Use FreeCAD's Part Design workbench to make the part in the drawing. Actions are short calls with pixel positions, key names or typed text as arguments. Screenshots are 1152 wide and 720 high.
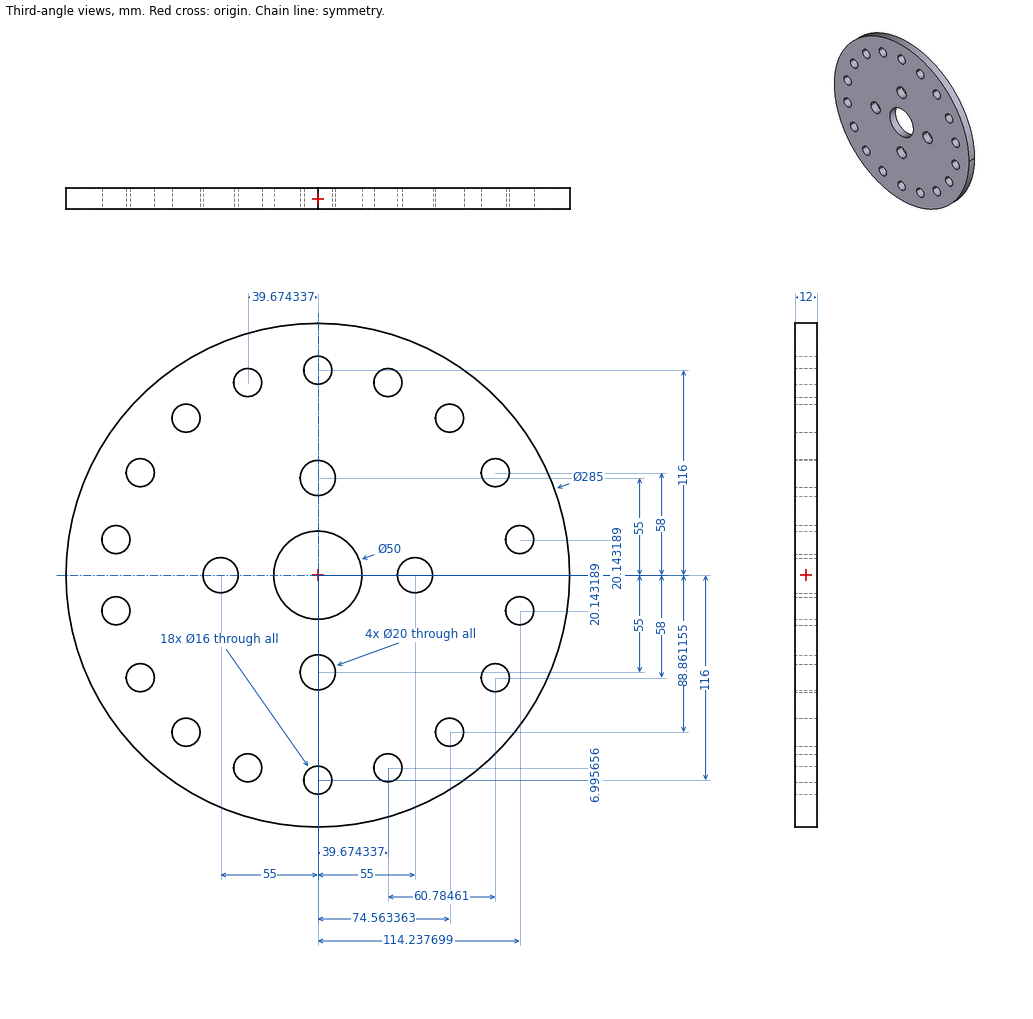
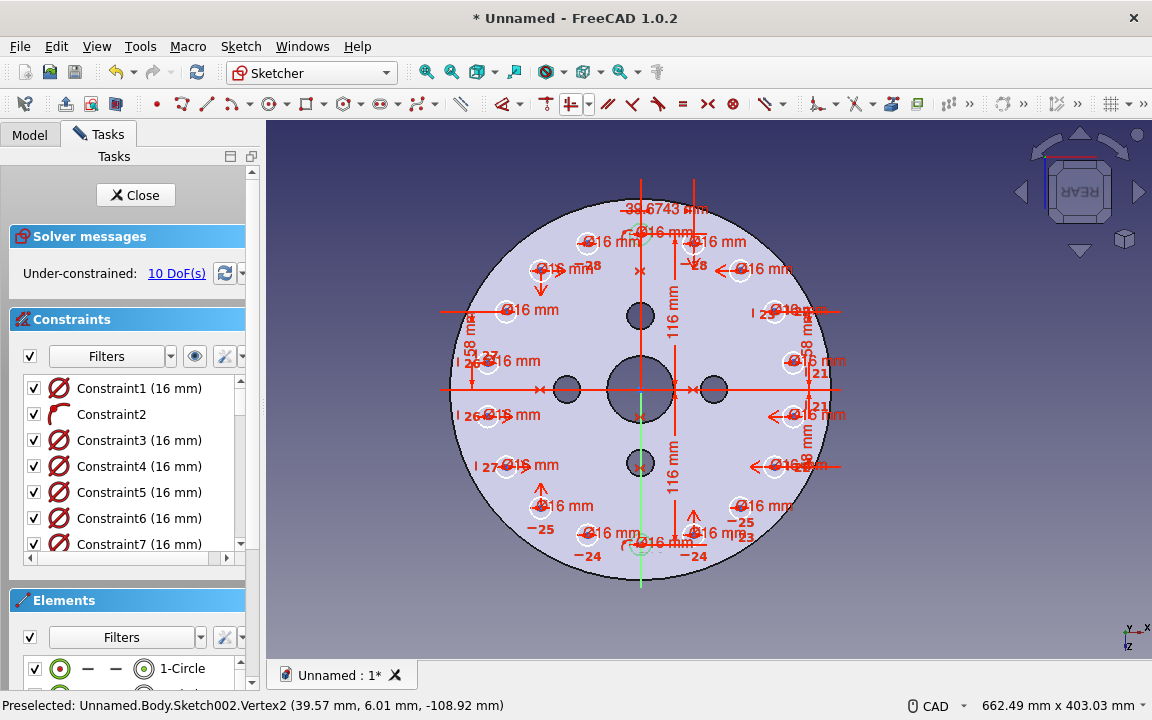
click(740, 271)
click(667, 237)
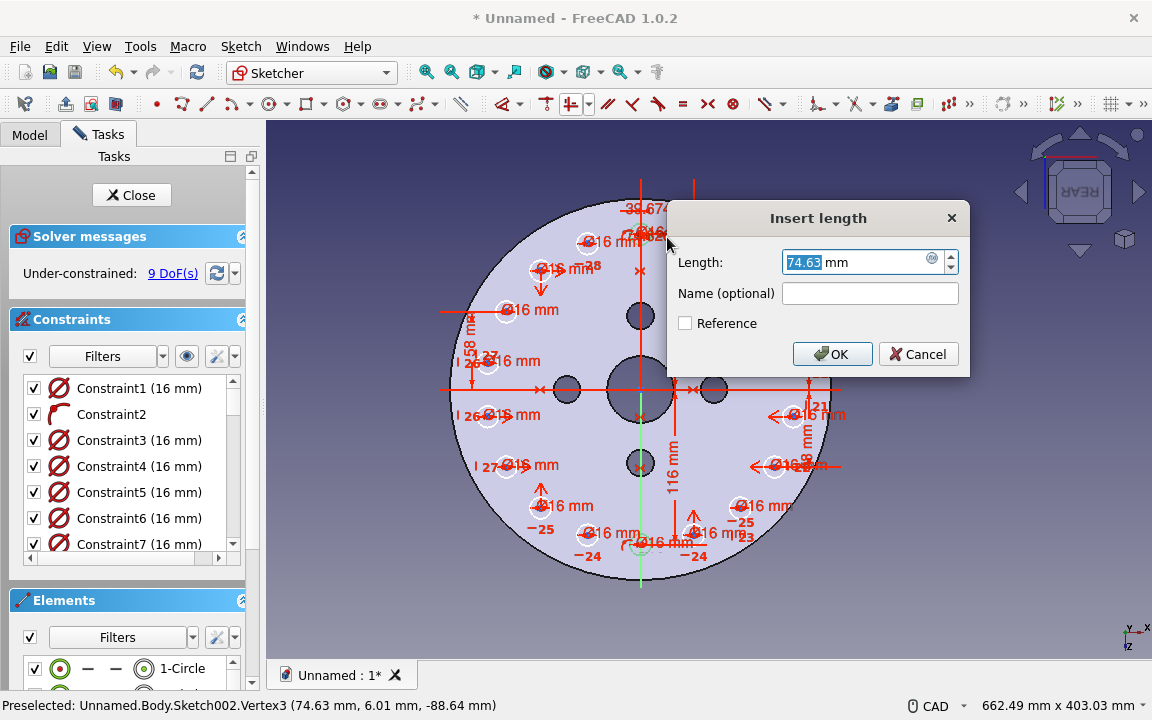
text(74.563363)
key(Return)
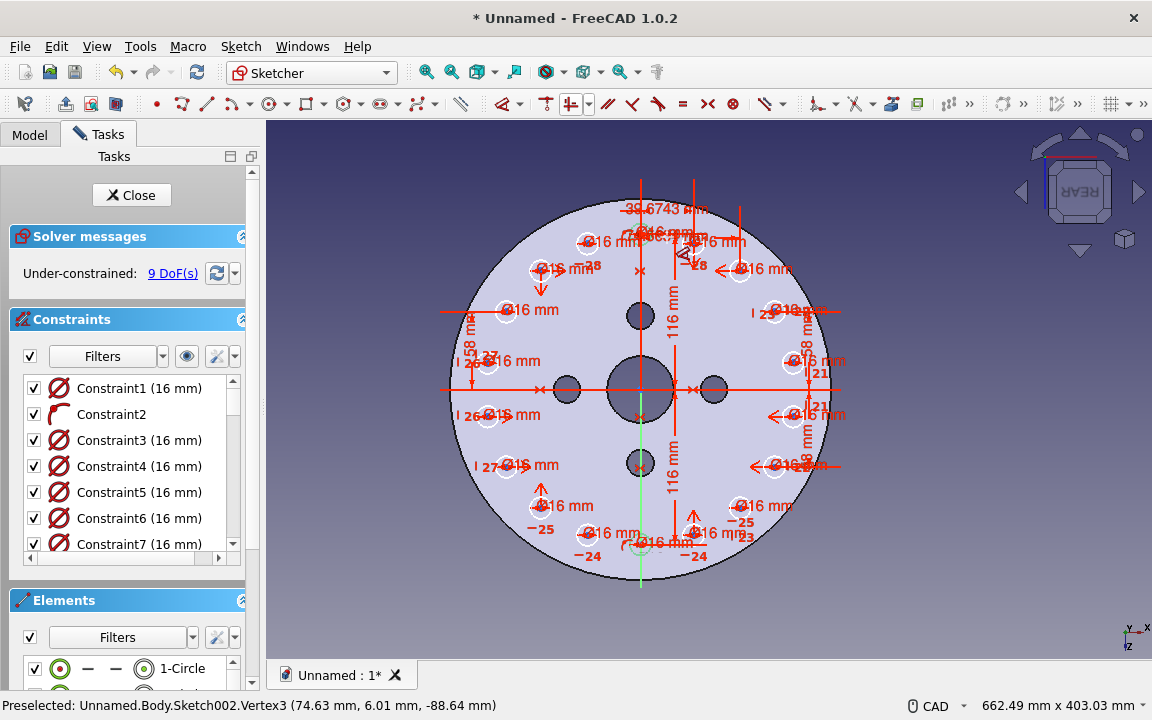
click(740, 271)
click(607, 357)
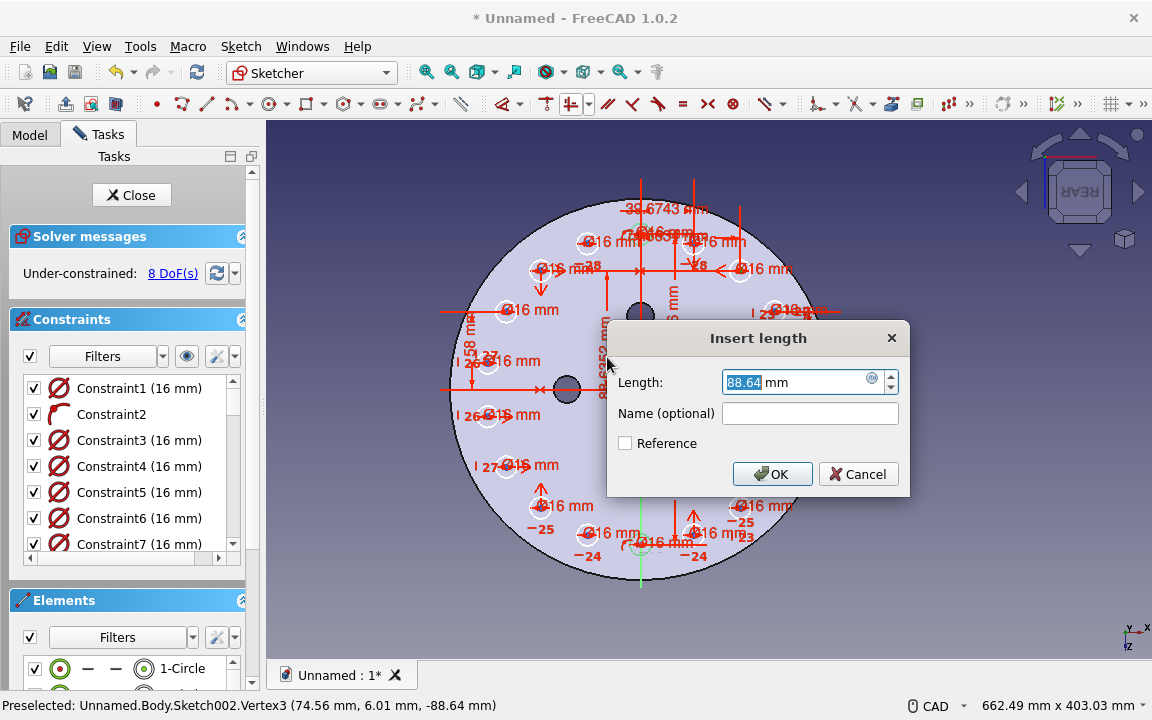
text(88.861155)
key(Return)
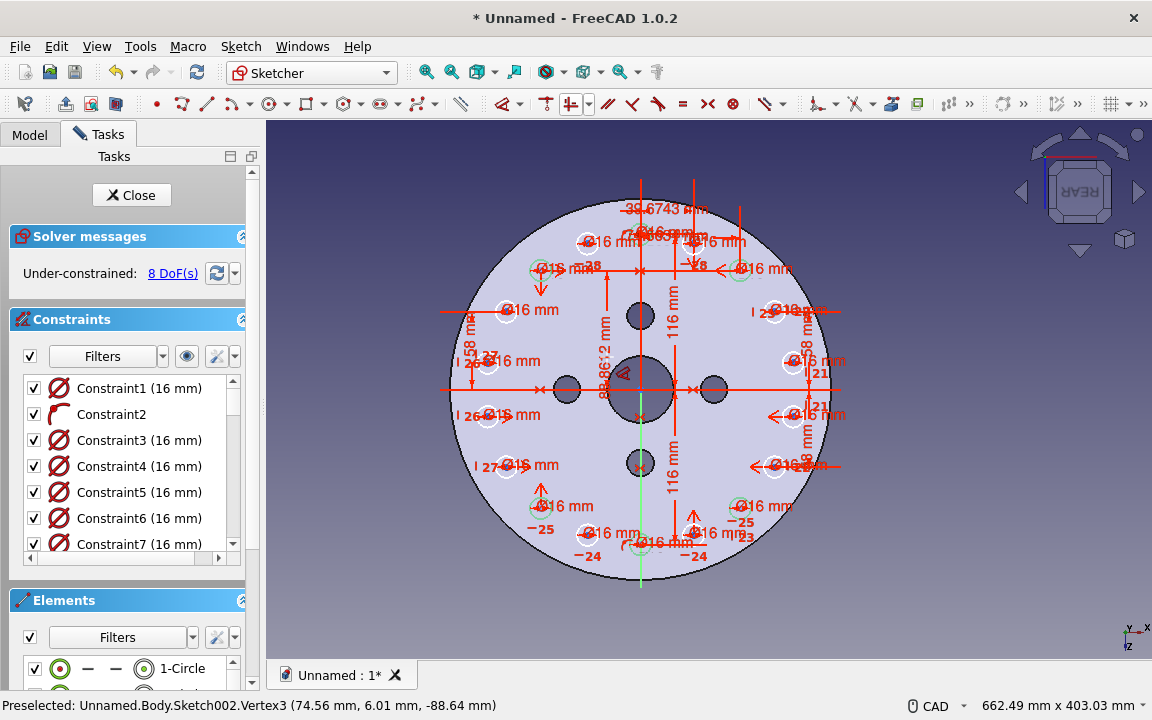
scroll(793, 363, up, 2)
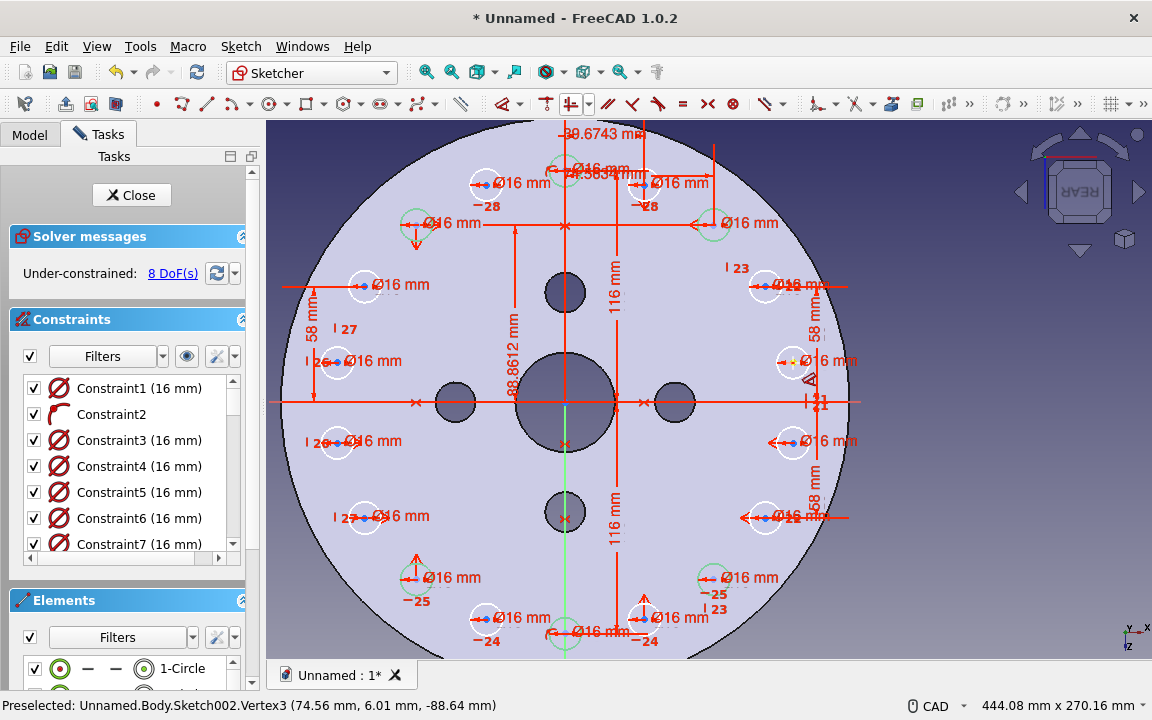
click(793, 363)
click(827, 383)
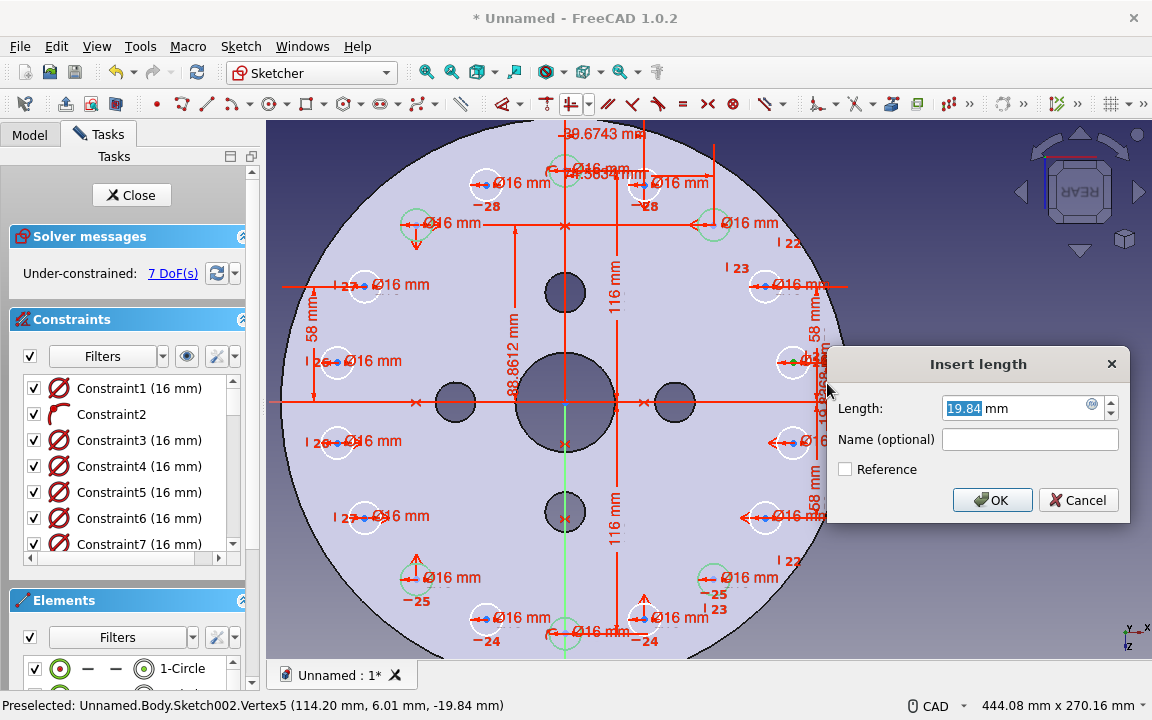
text(20.143189)
key(Return)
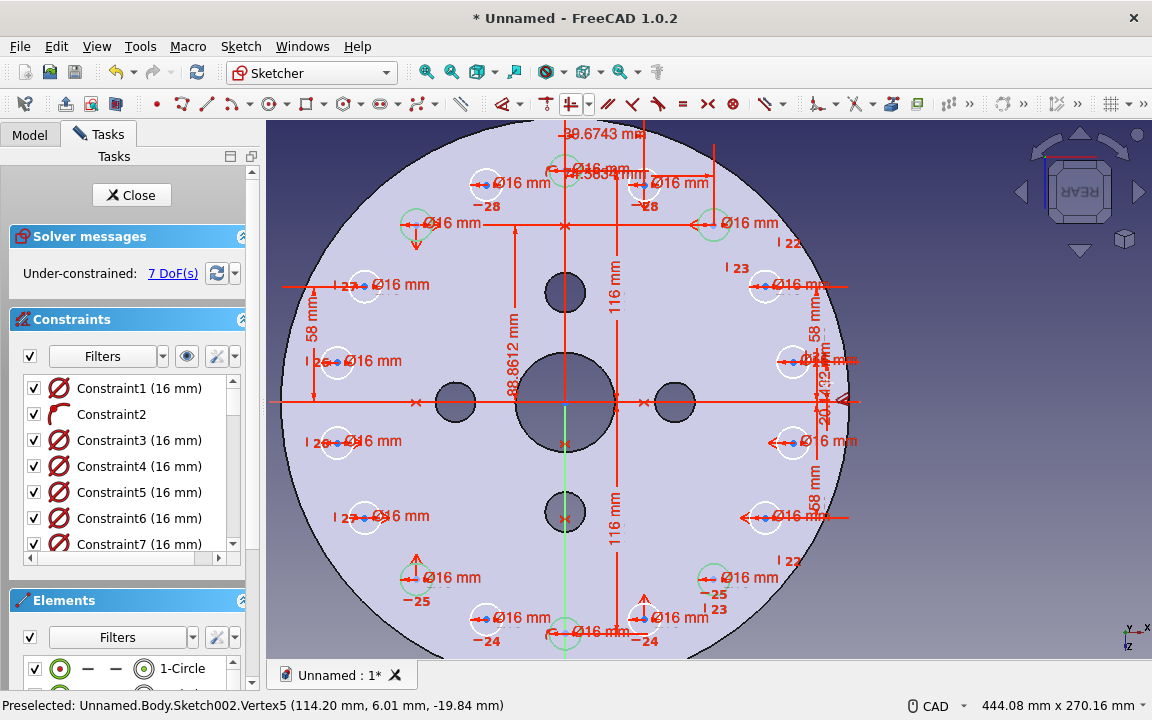
click(793, 443)
click(827, 423)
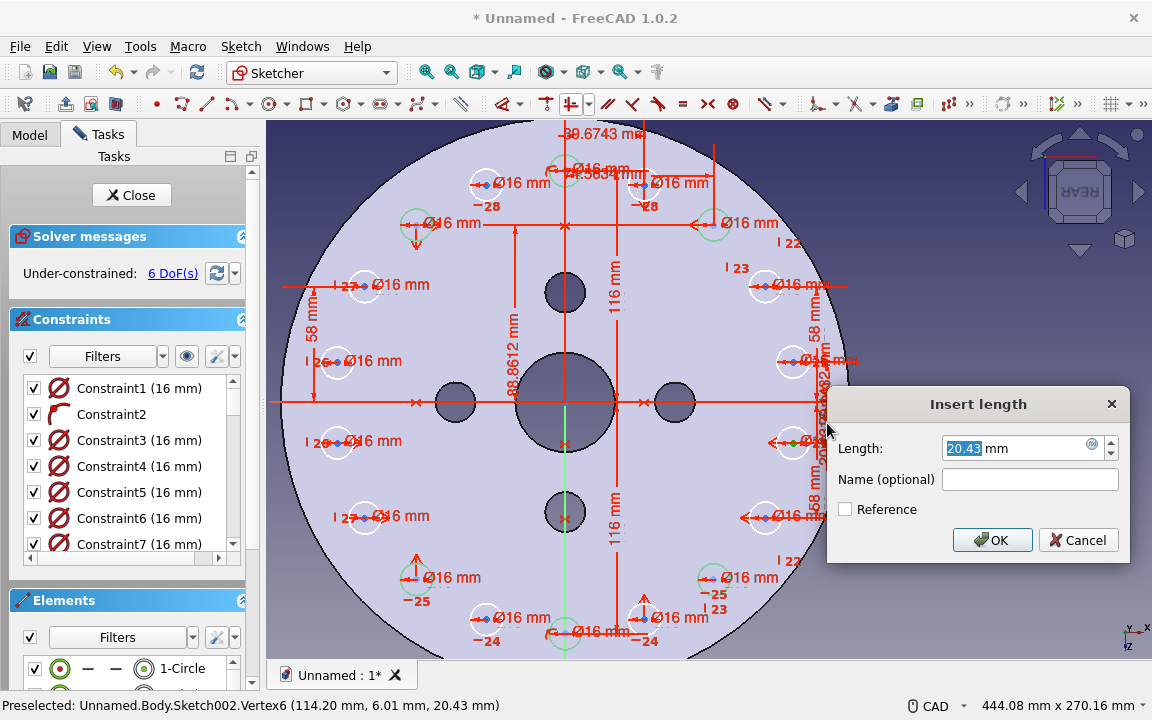
text(20.143189)
key(Return)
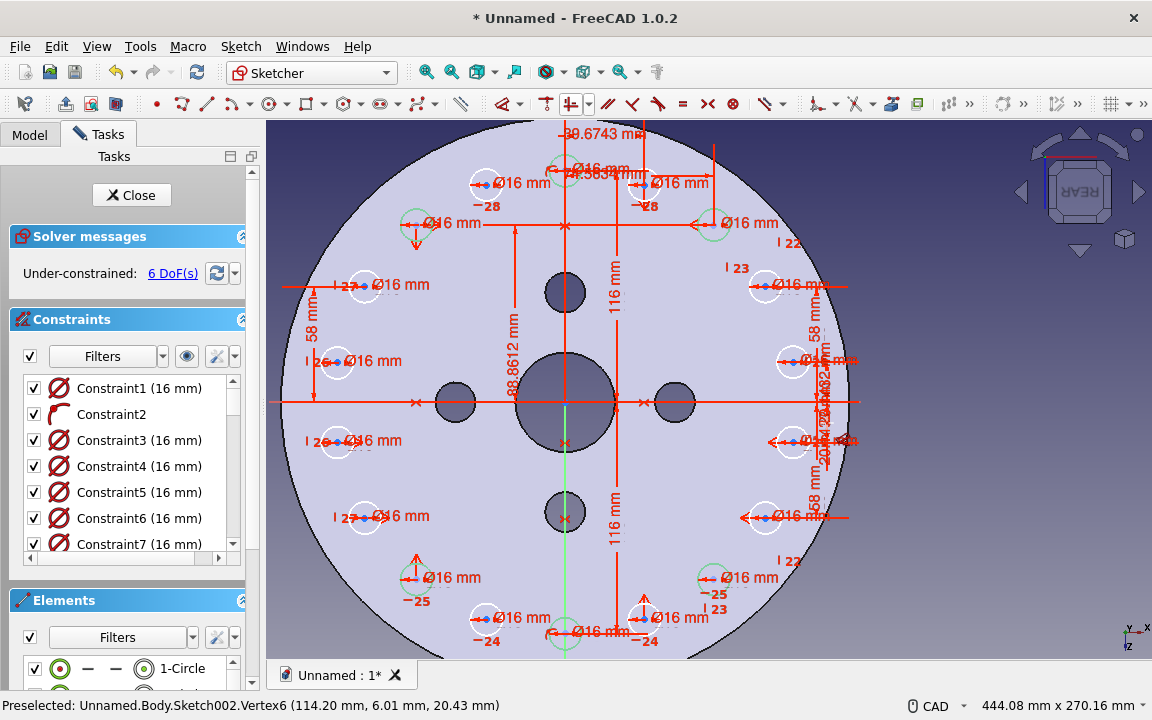
click(486, 620)
click(526, 320)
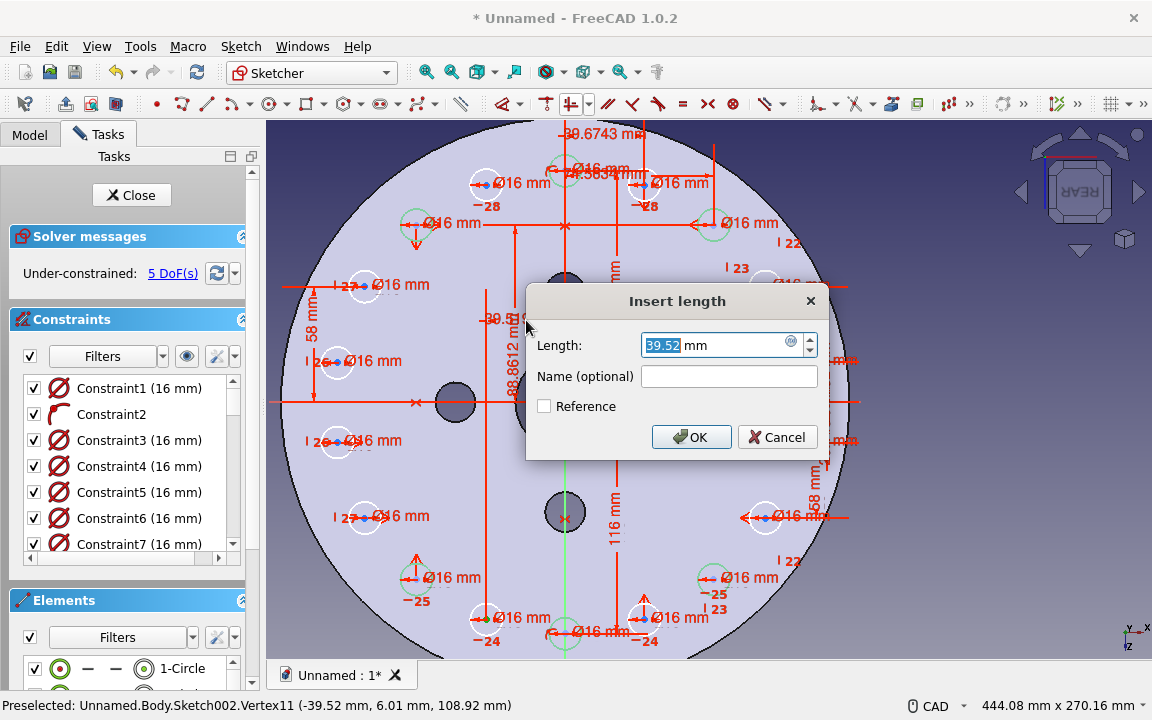
text(39.674337)
key(Return)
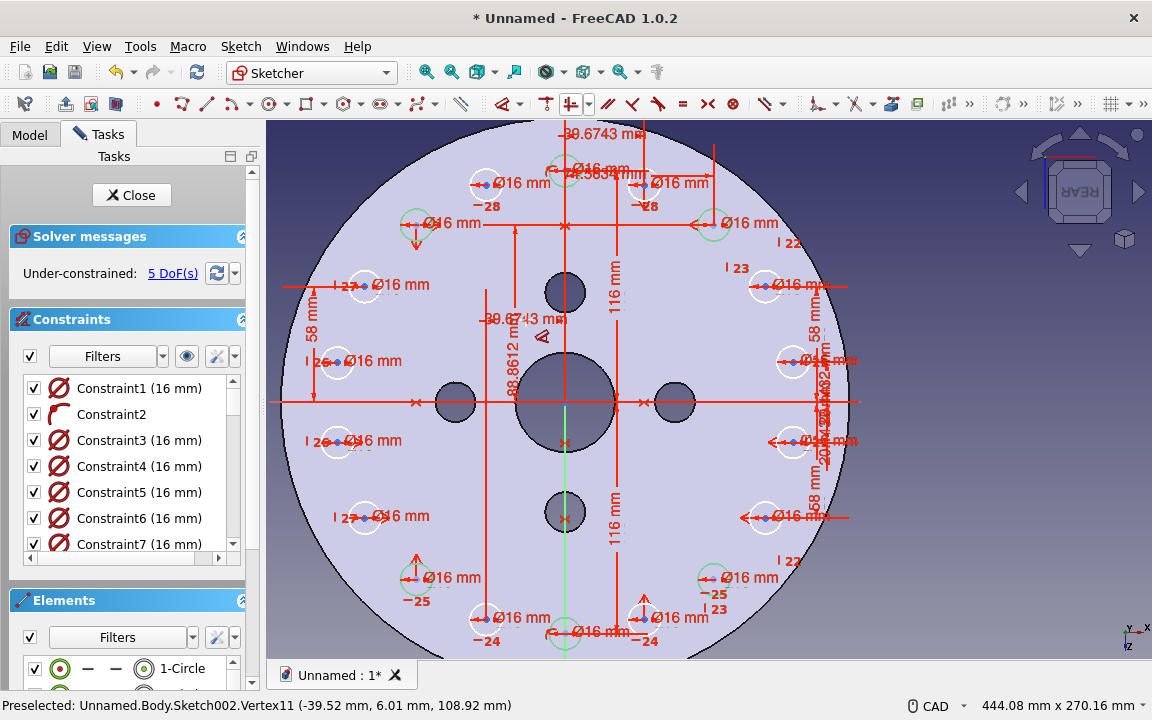
click(337, 363)
click(303, 383)